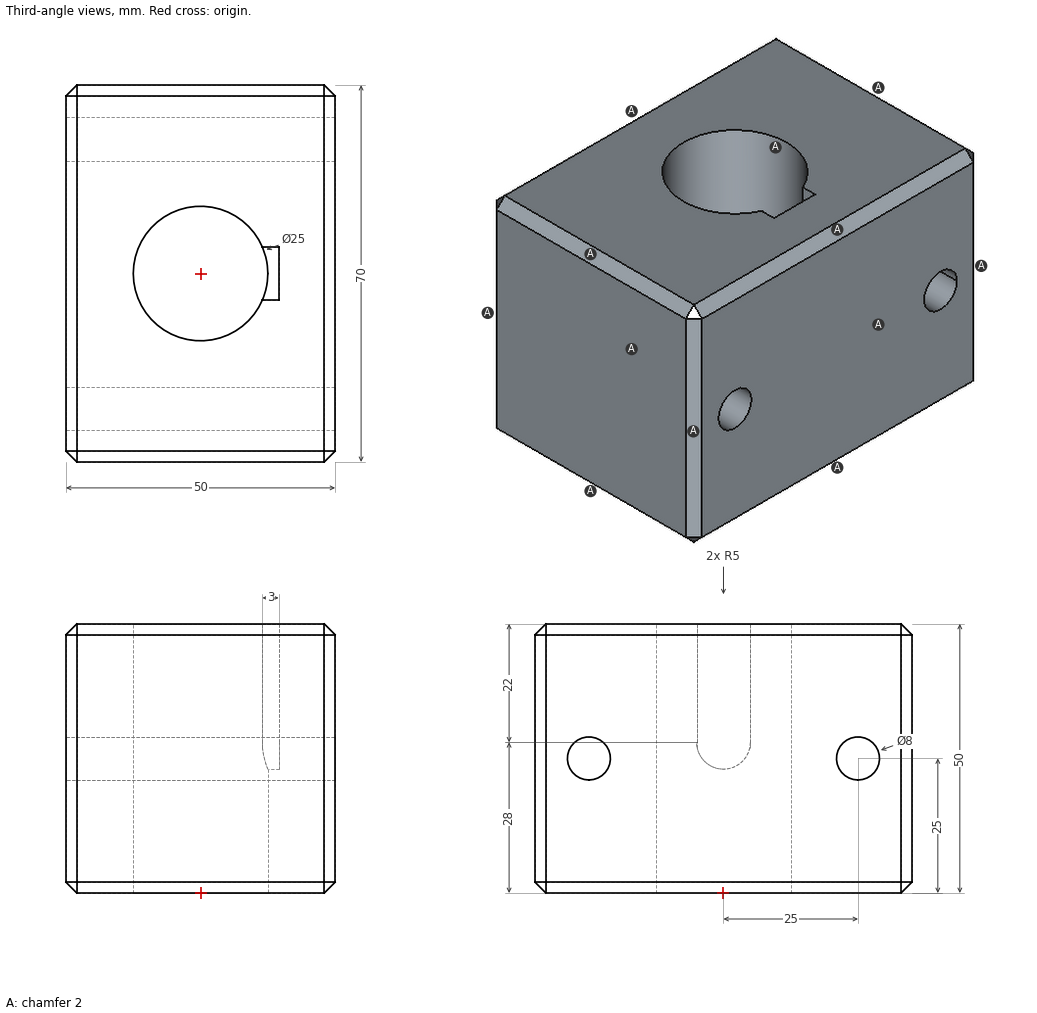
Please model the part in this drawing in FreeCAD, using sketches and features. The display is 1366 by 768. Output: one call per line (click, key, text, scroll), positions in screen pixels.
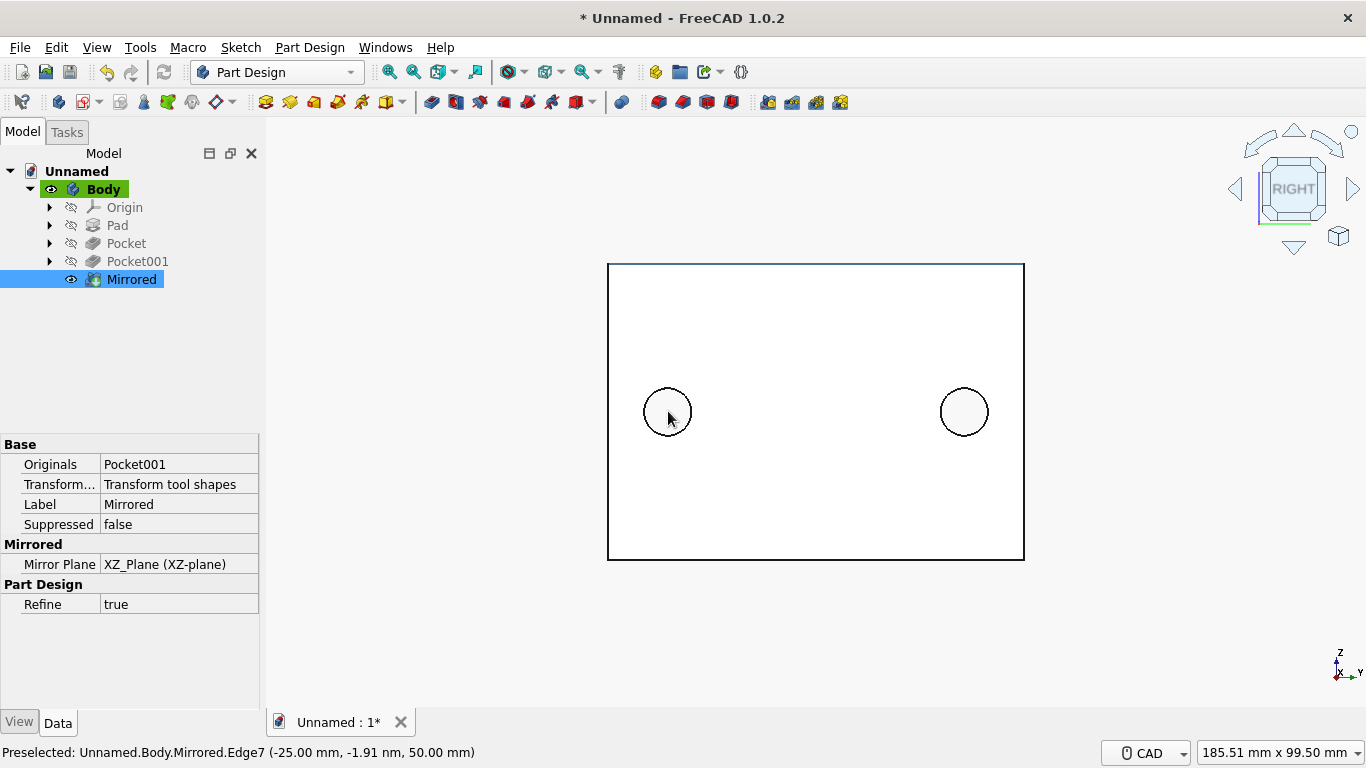
click(816, 559, ctrl)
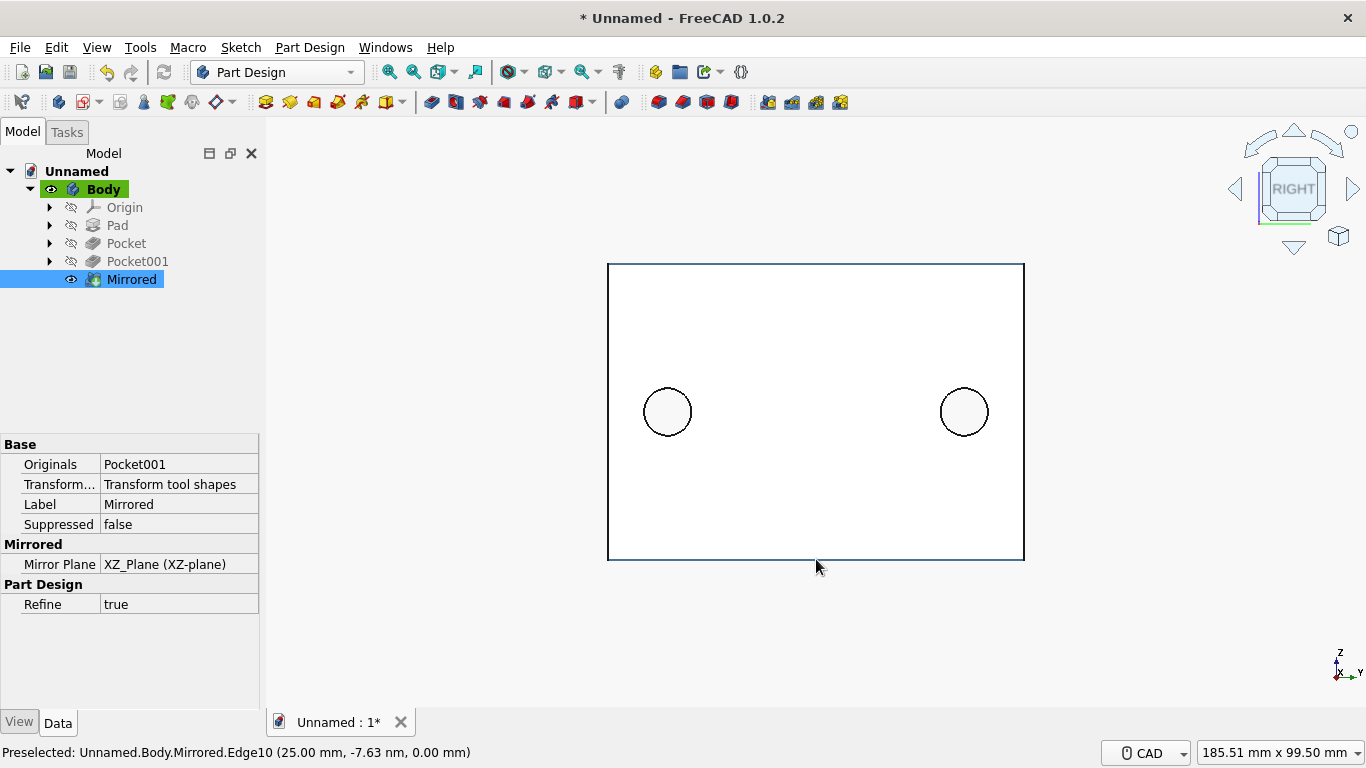
key(5)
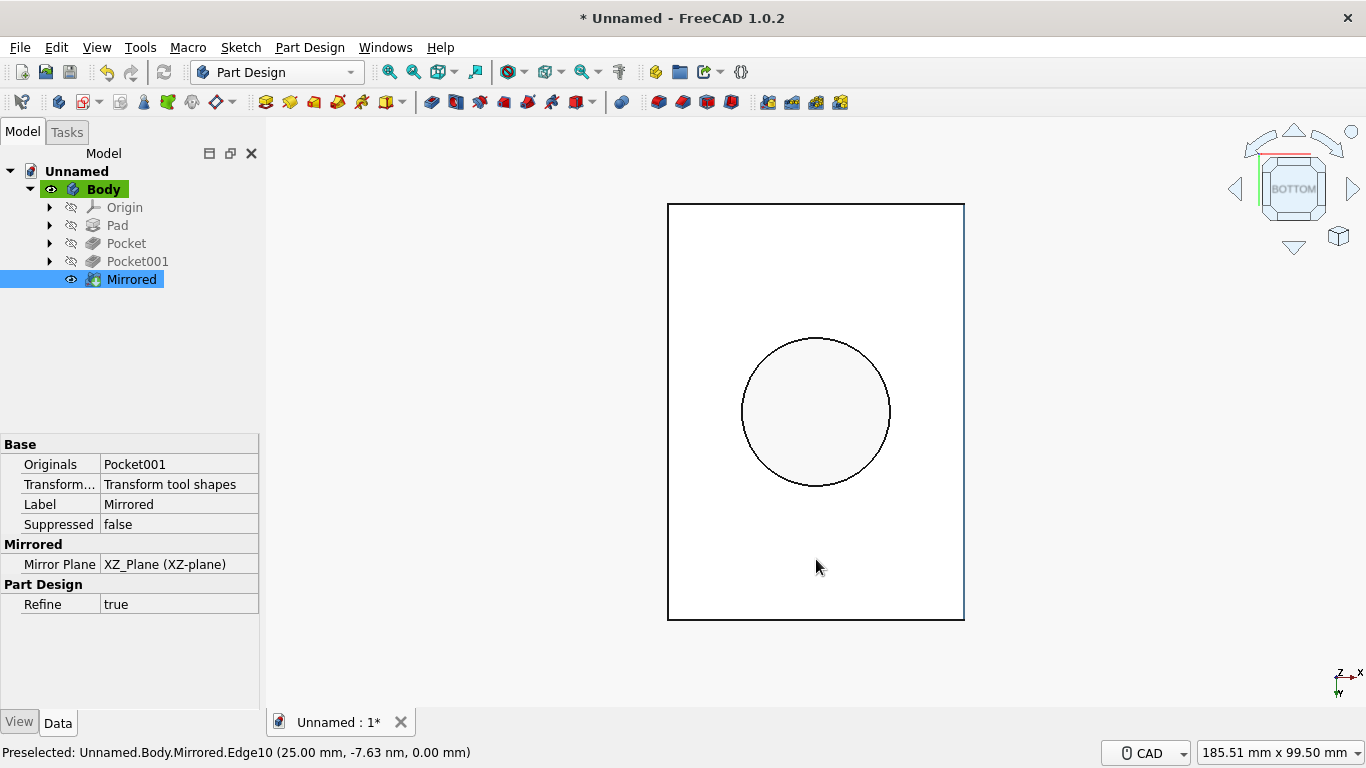
click(668, 411, ctrl)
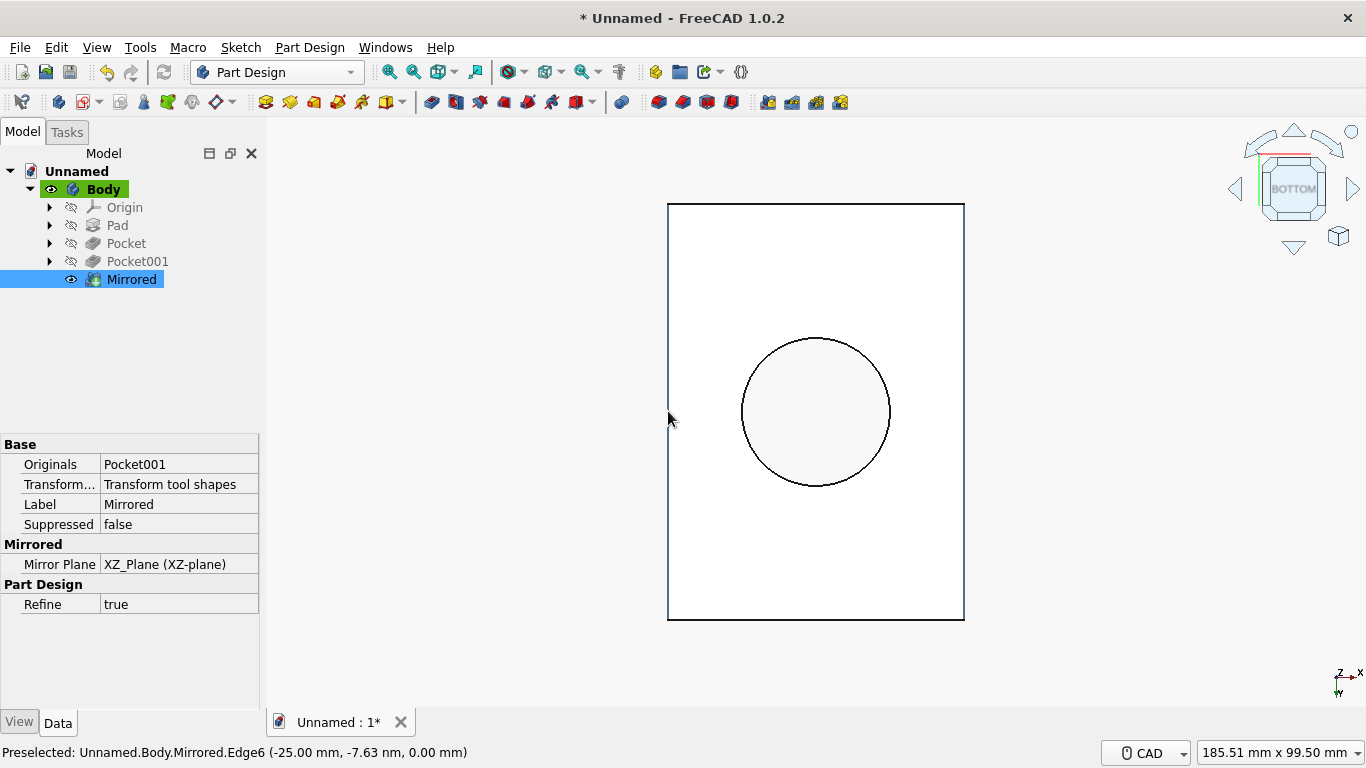
key(4)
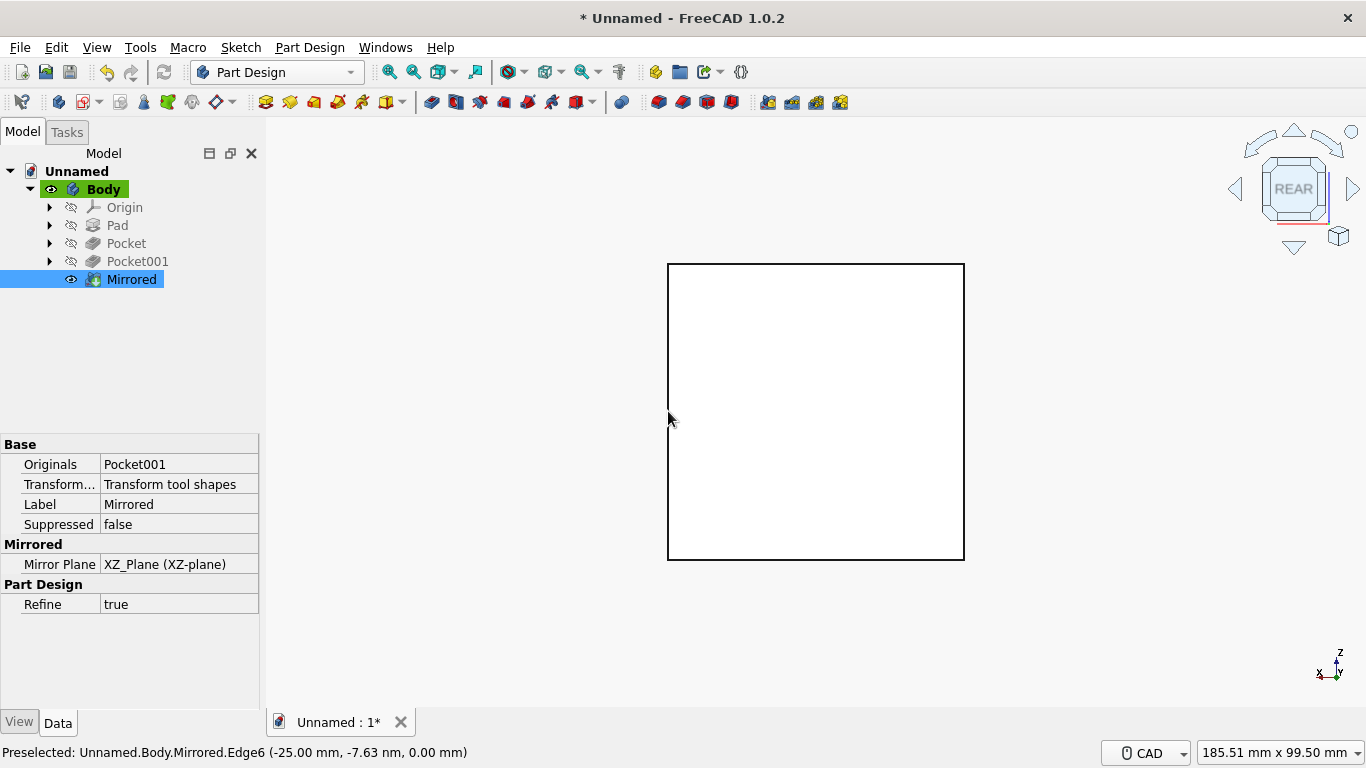
click(816, 411, ctrl)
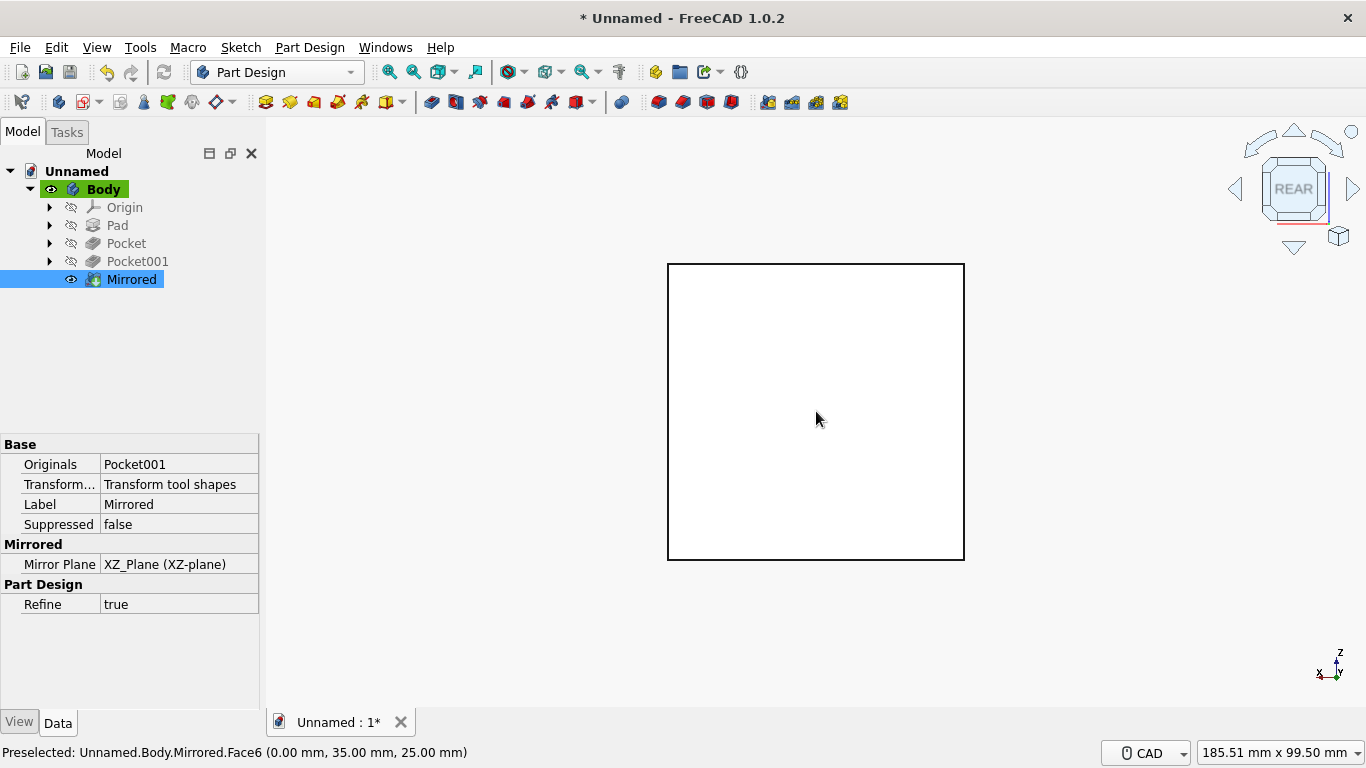
click(684, 102)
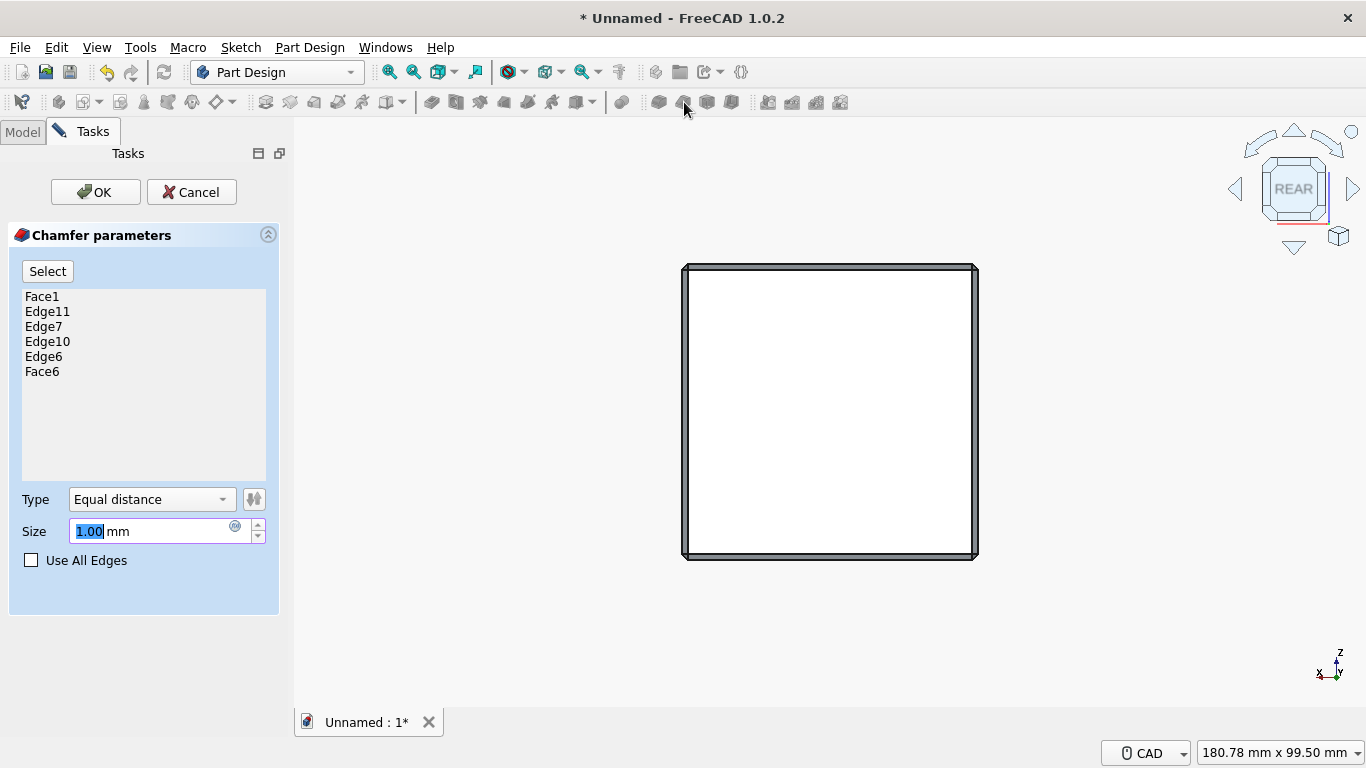
text(2)
key(Tab)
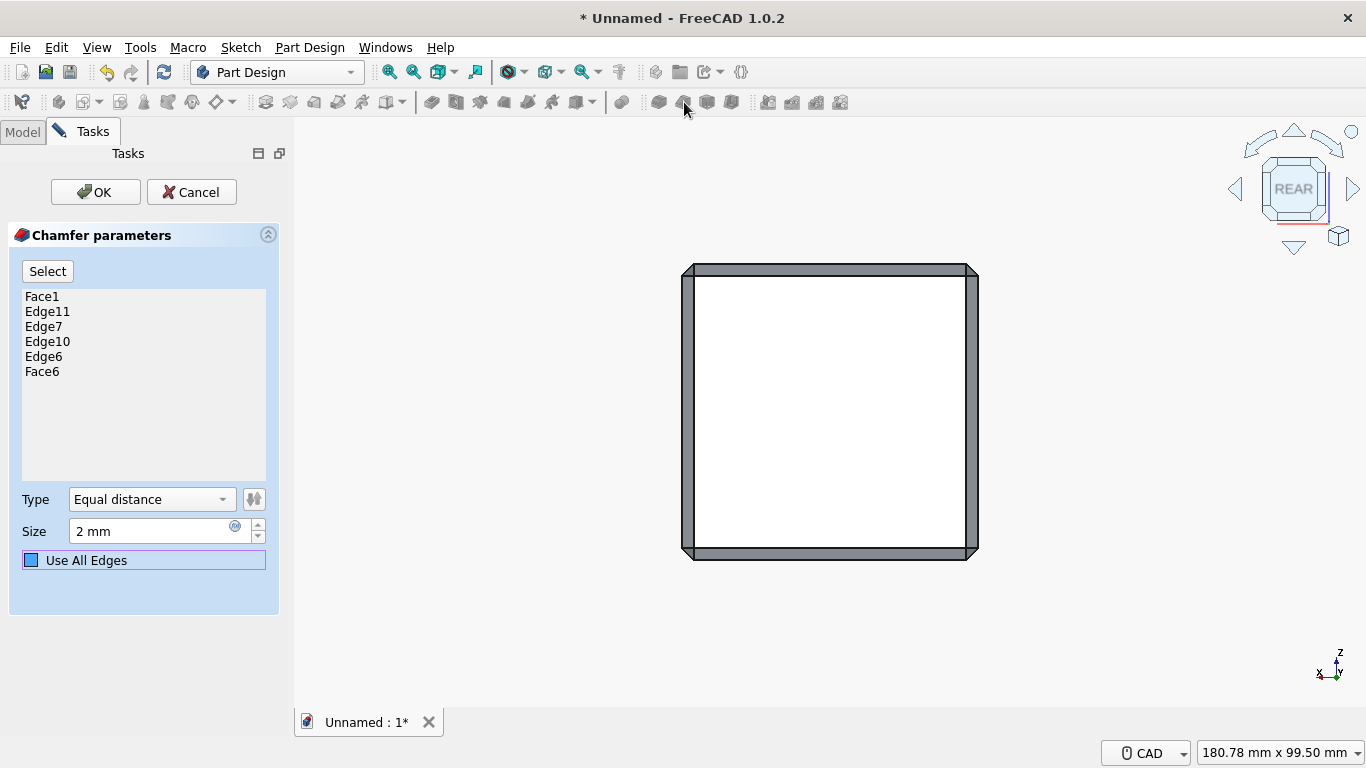
click(96, 192)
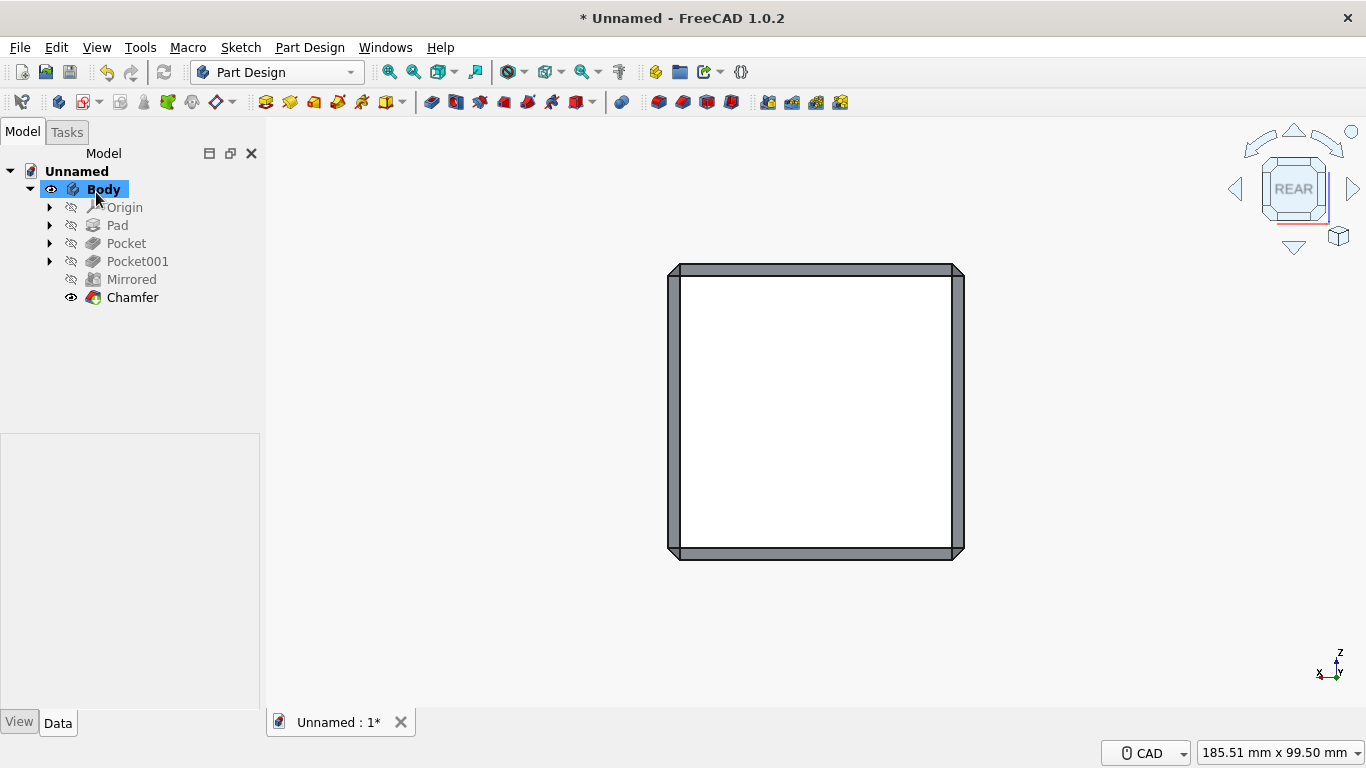
click(50, 207)